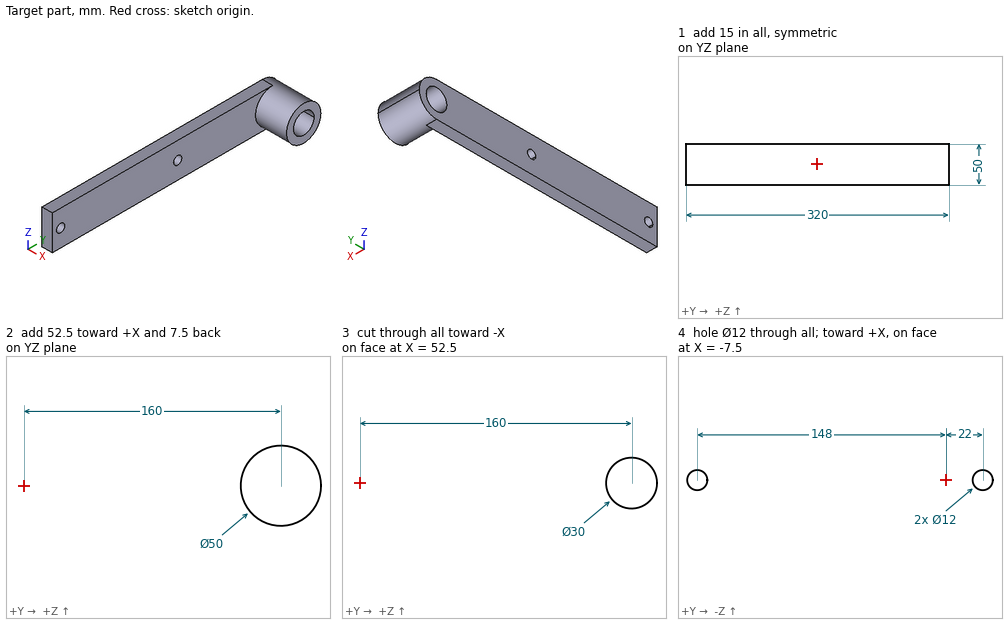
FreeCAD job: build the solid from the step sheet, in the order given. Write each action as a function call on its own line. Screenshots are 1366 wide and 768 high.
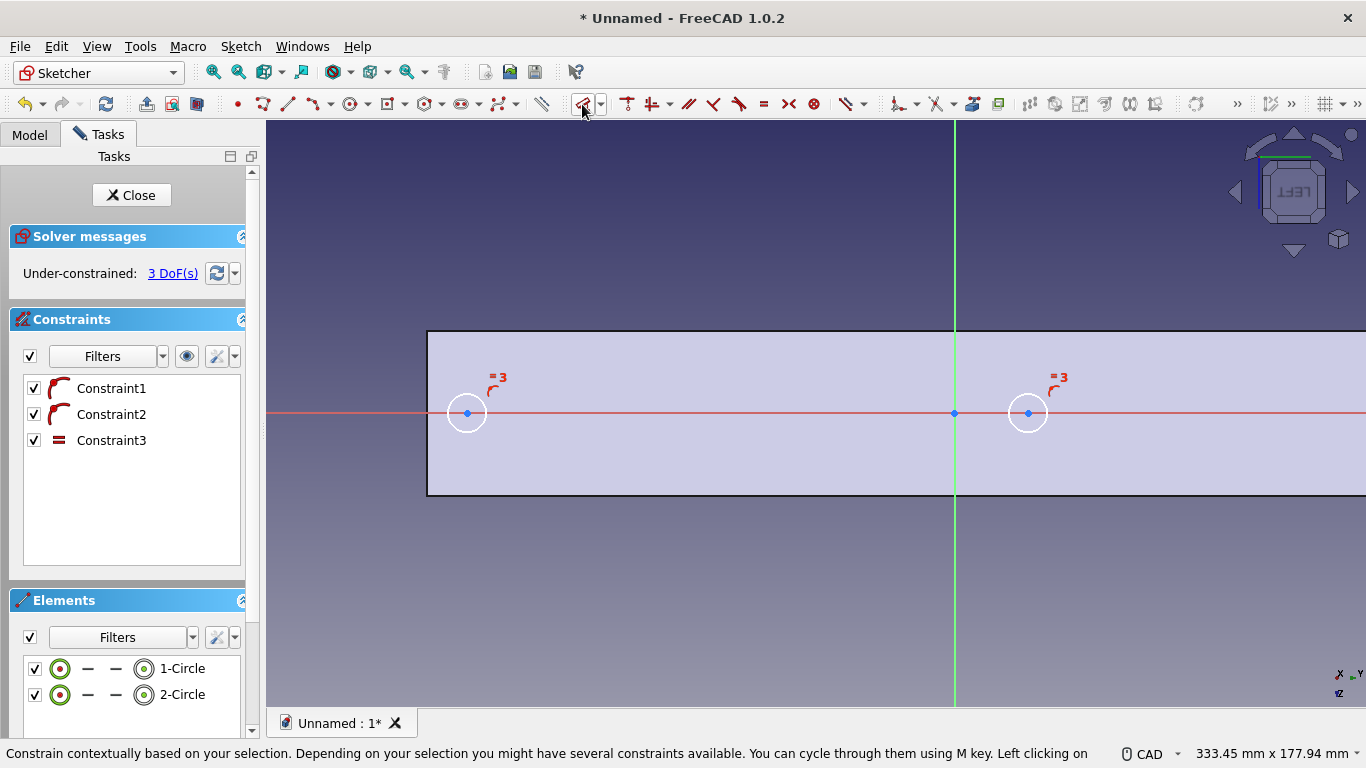
click(1041, 400)
click(1064, 377)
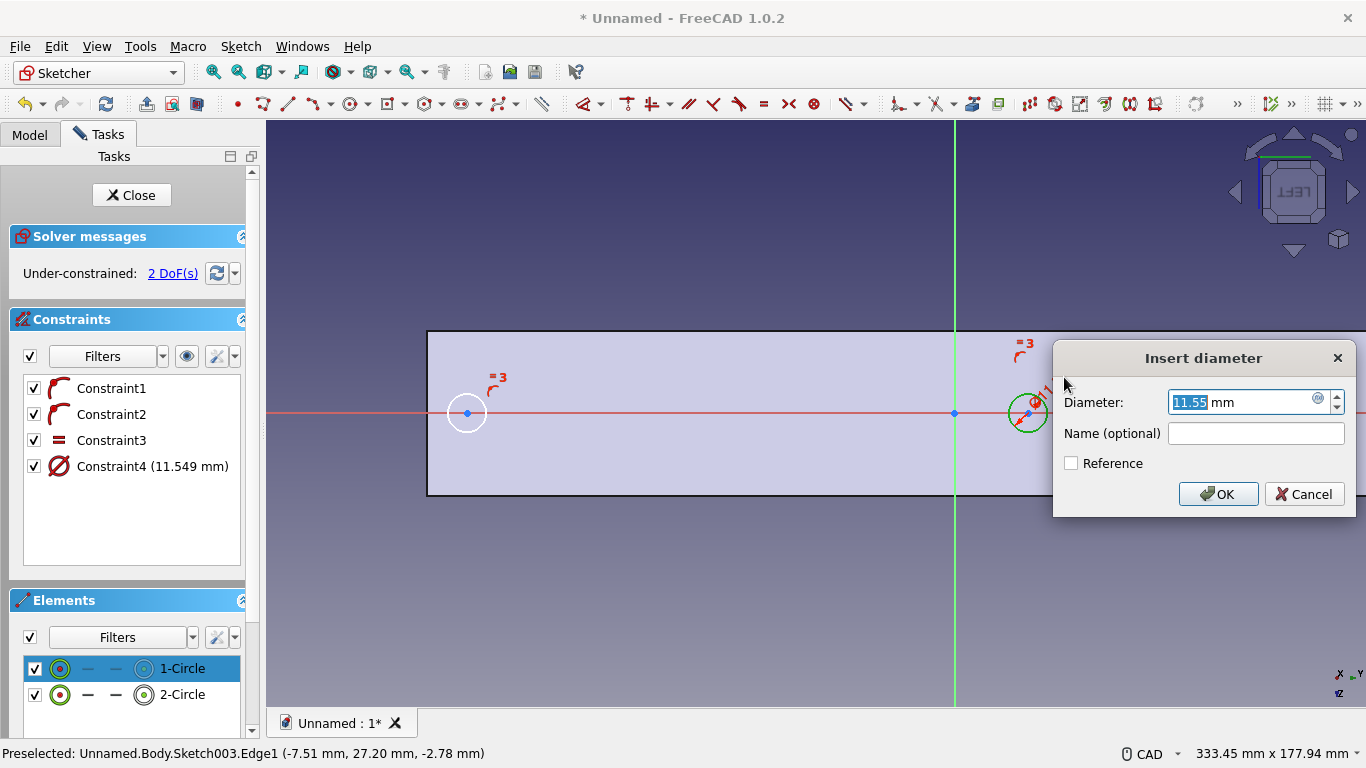
text(12)
key(Return)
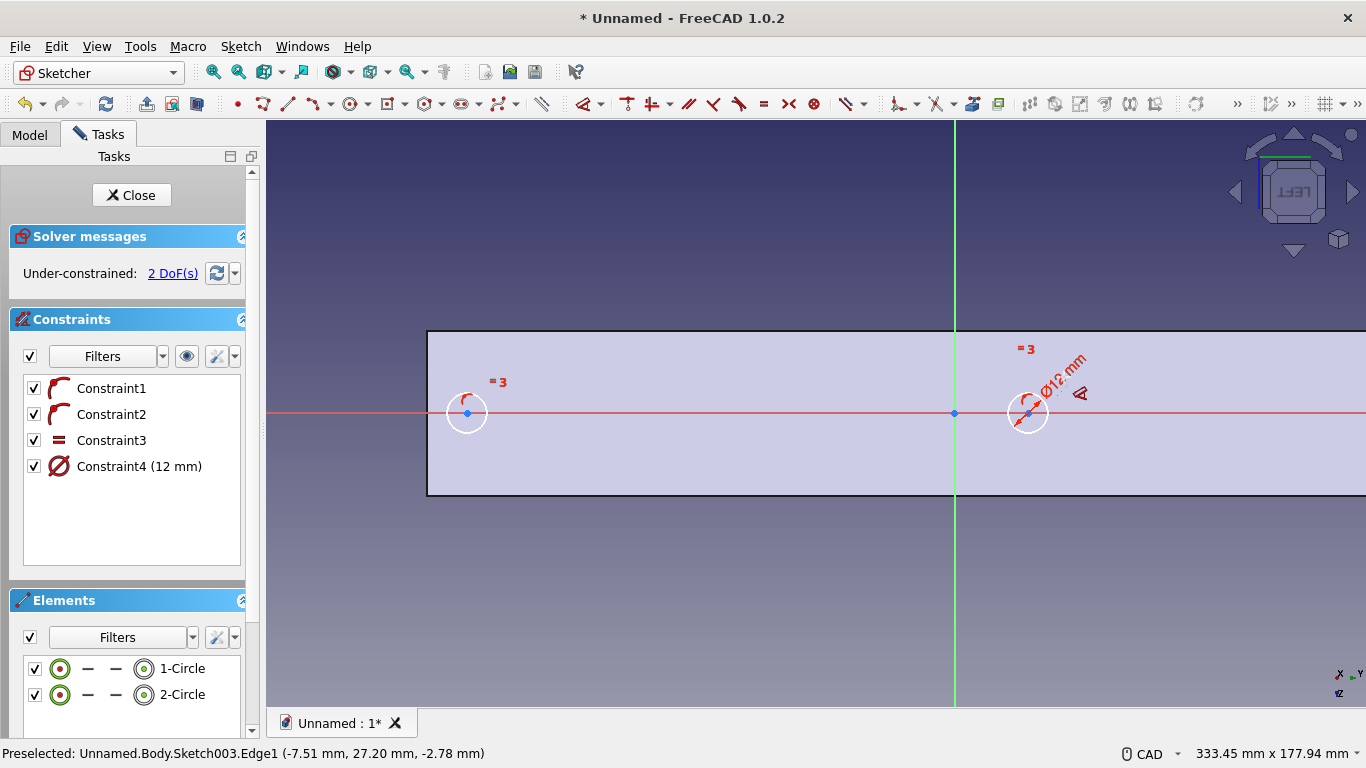
click(1028, 413)
click(991, 447)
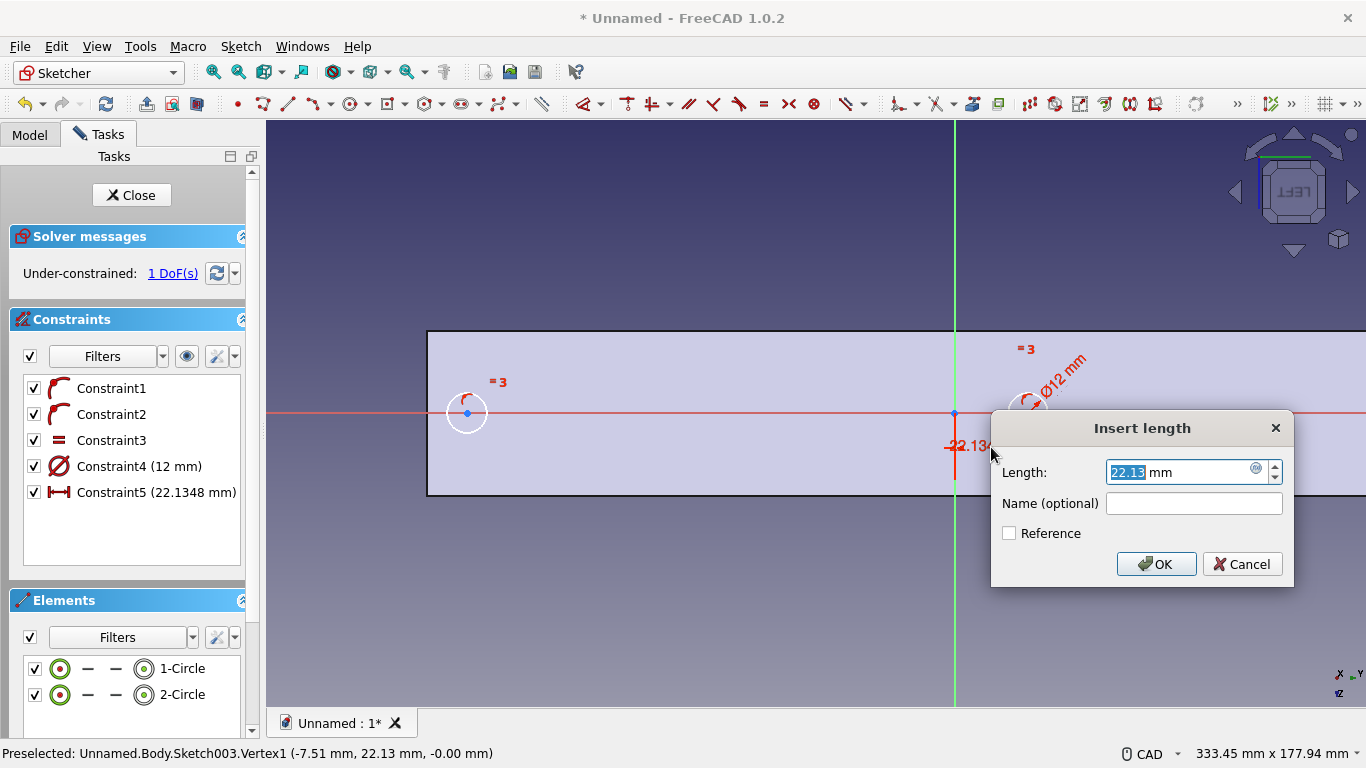
text(22)
key(Return)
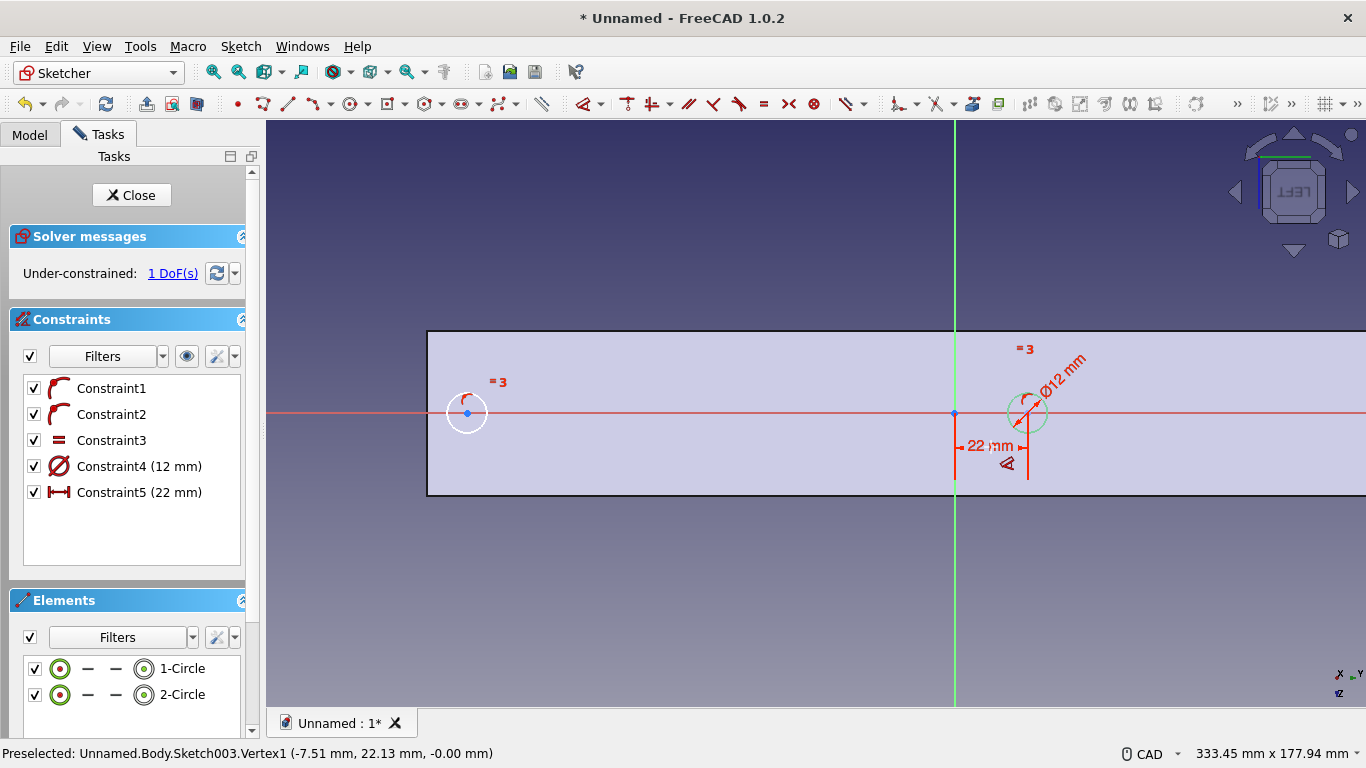
click(467, 413)
click(711, 447)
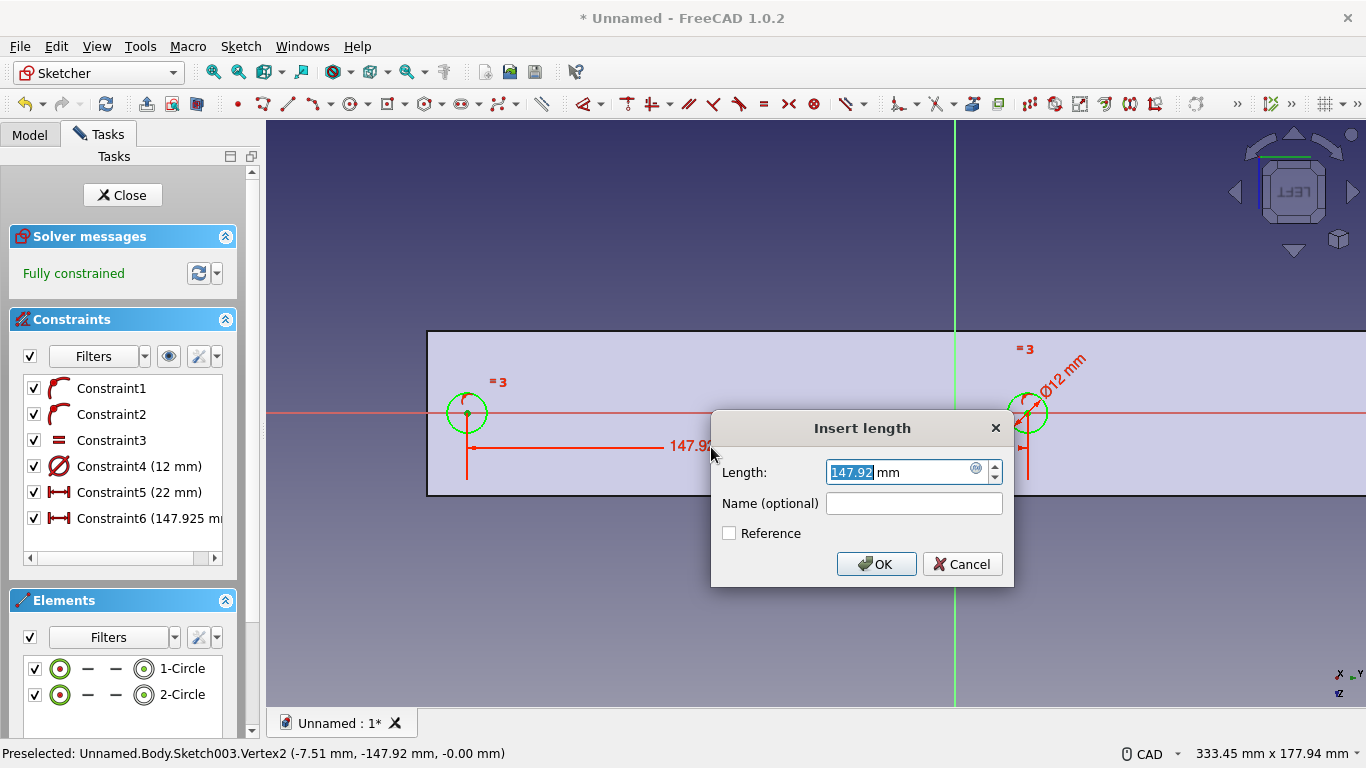
text(148)
key(Return)
key(Escape)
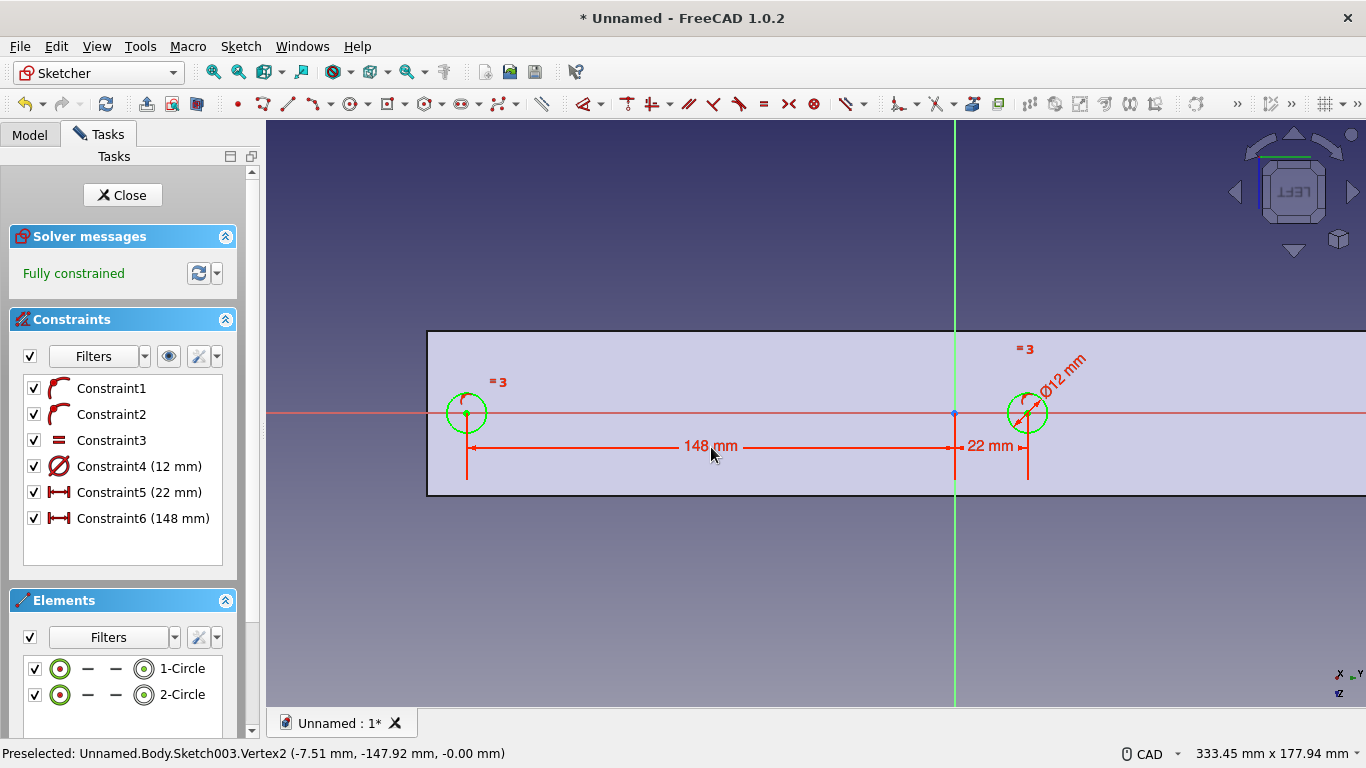
click(123, 195)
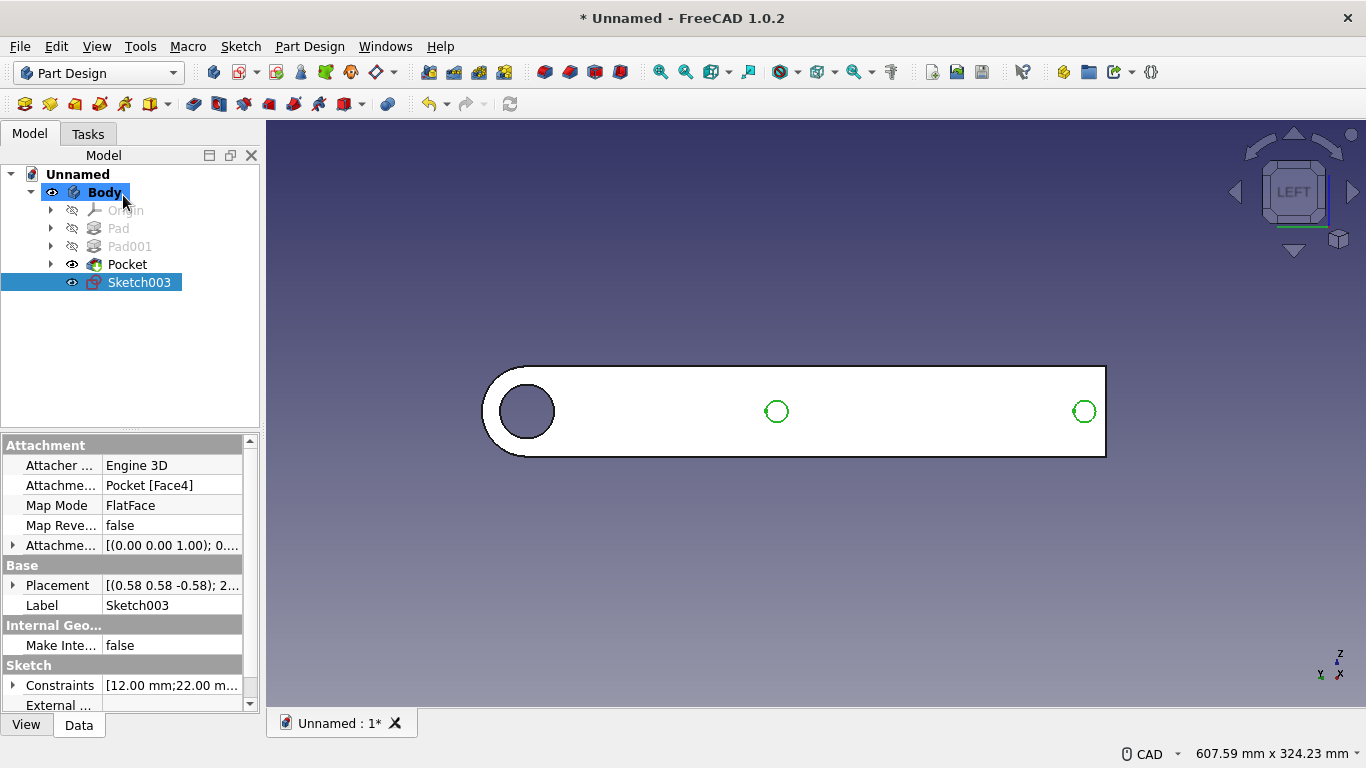
click(219, 104)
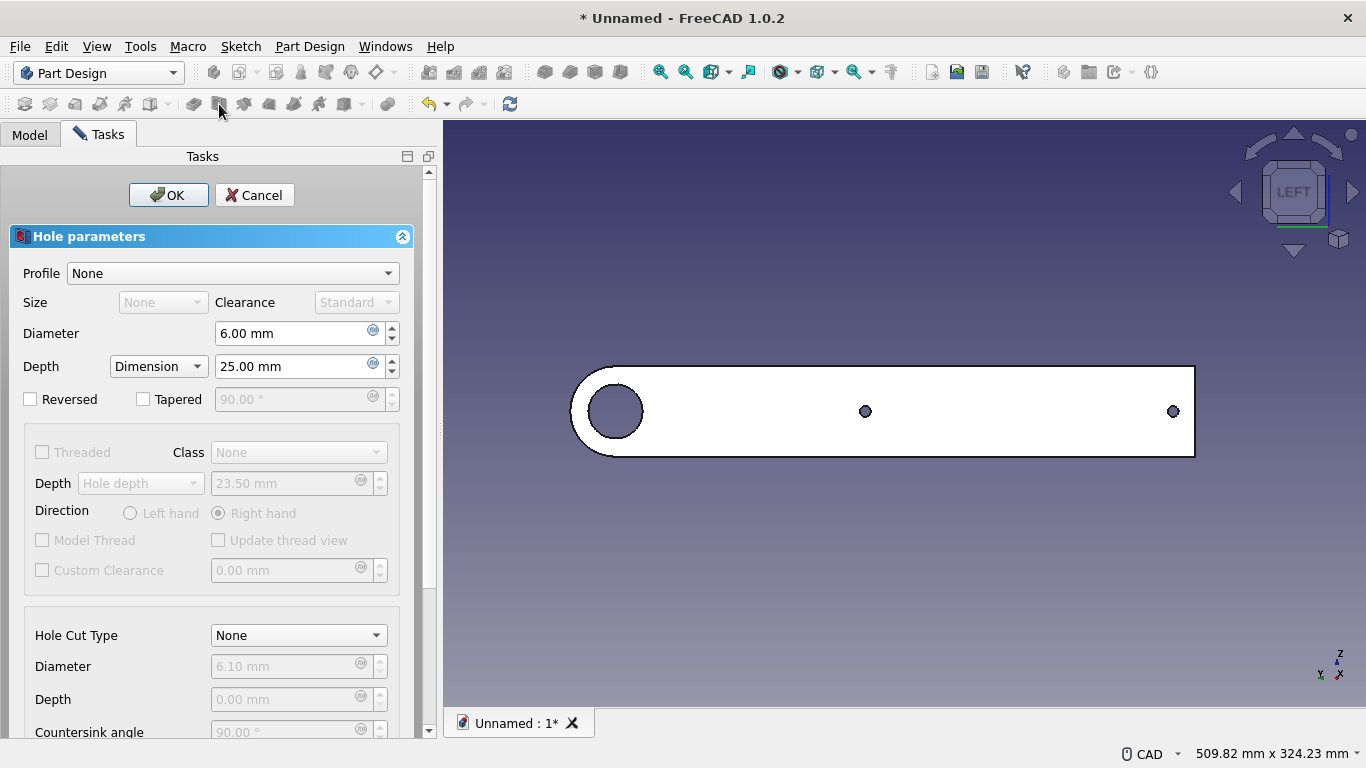
triple_click(300, 334)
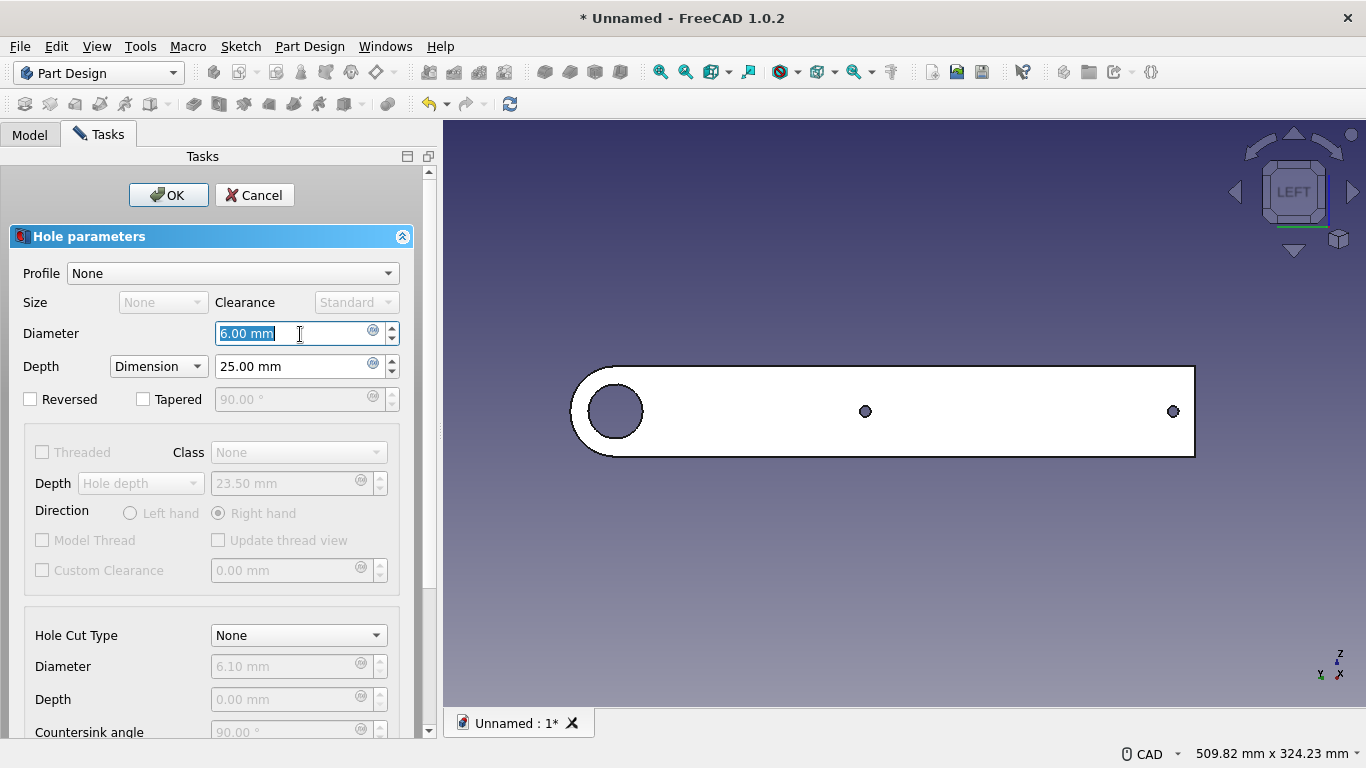
text(12)
key(Tab)